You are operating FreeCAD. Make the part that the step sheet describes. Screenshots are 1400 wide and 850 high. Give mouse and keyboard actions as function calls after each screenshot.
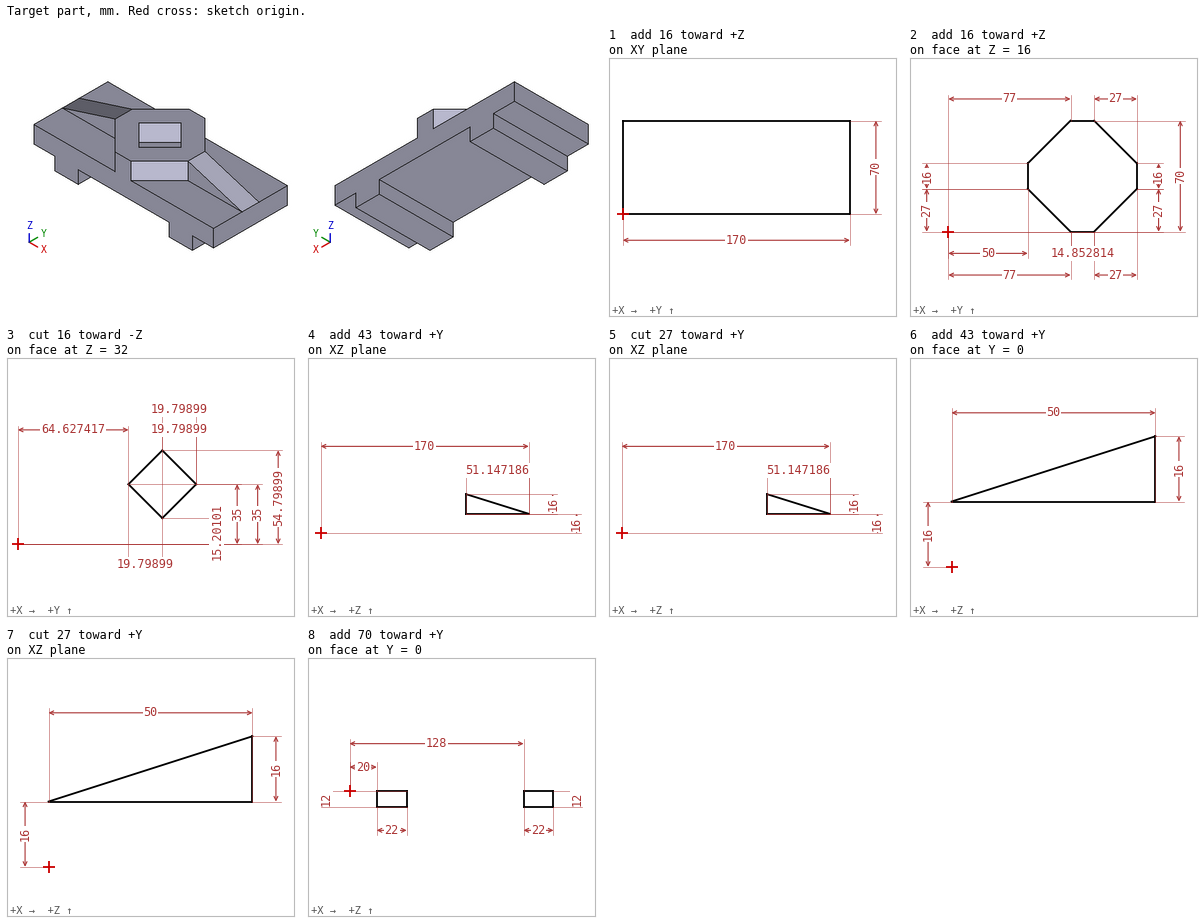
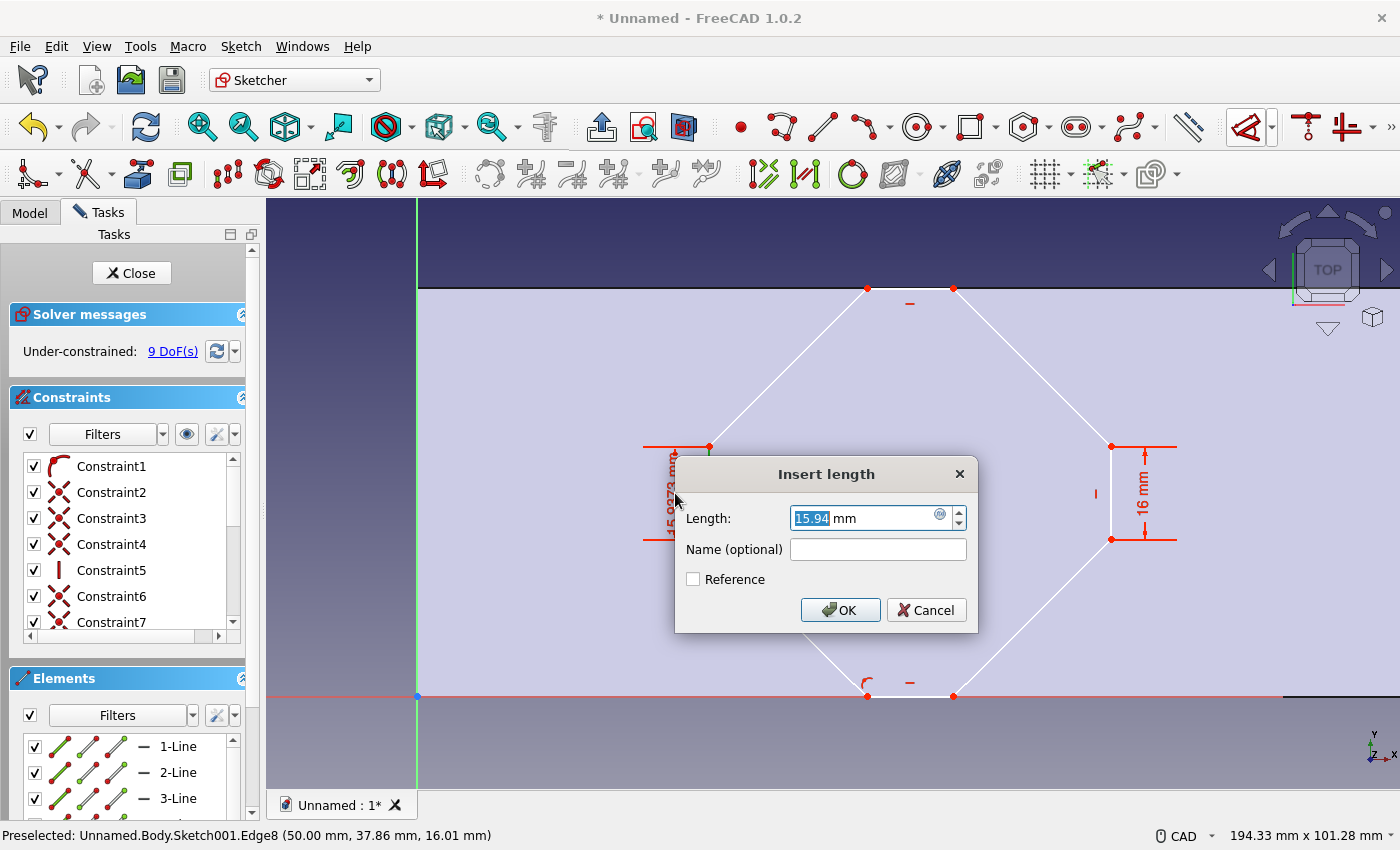
text(16)
key(Return)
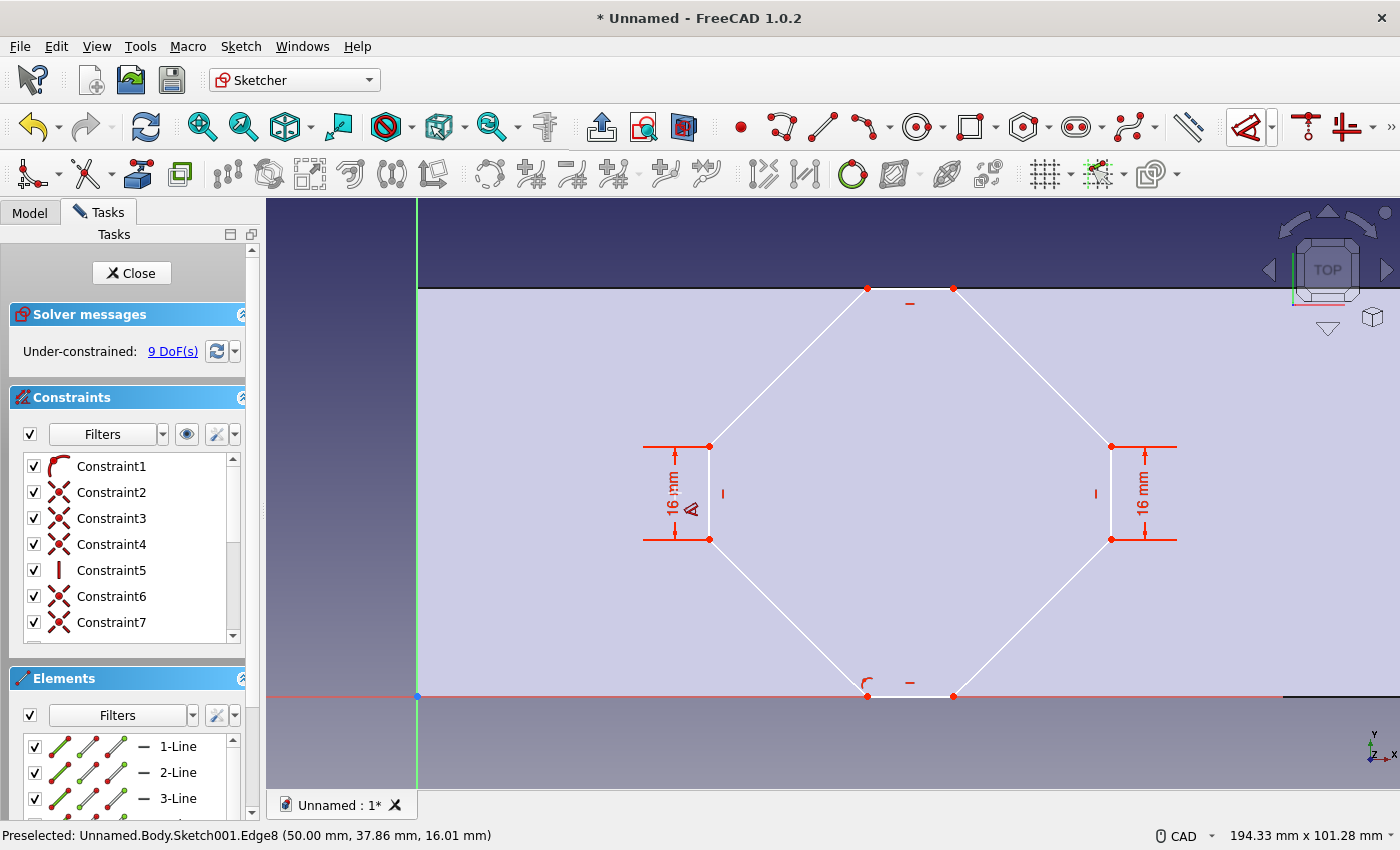
click(709, 540)
click(563, 731)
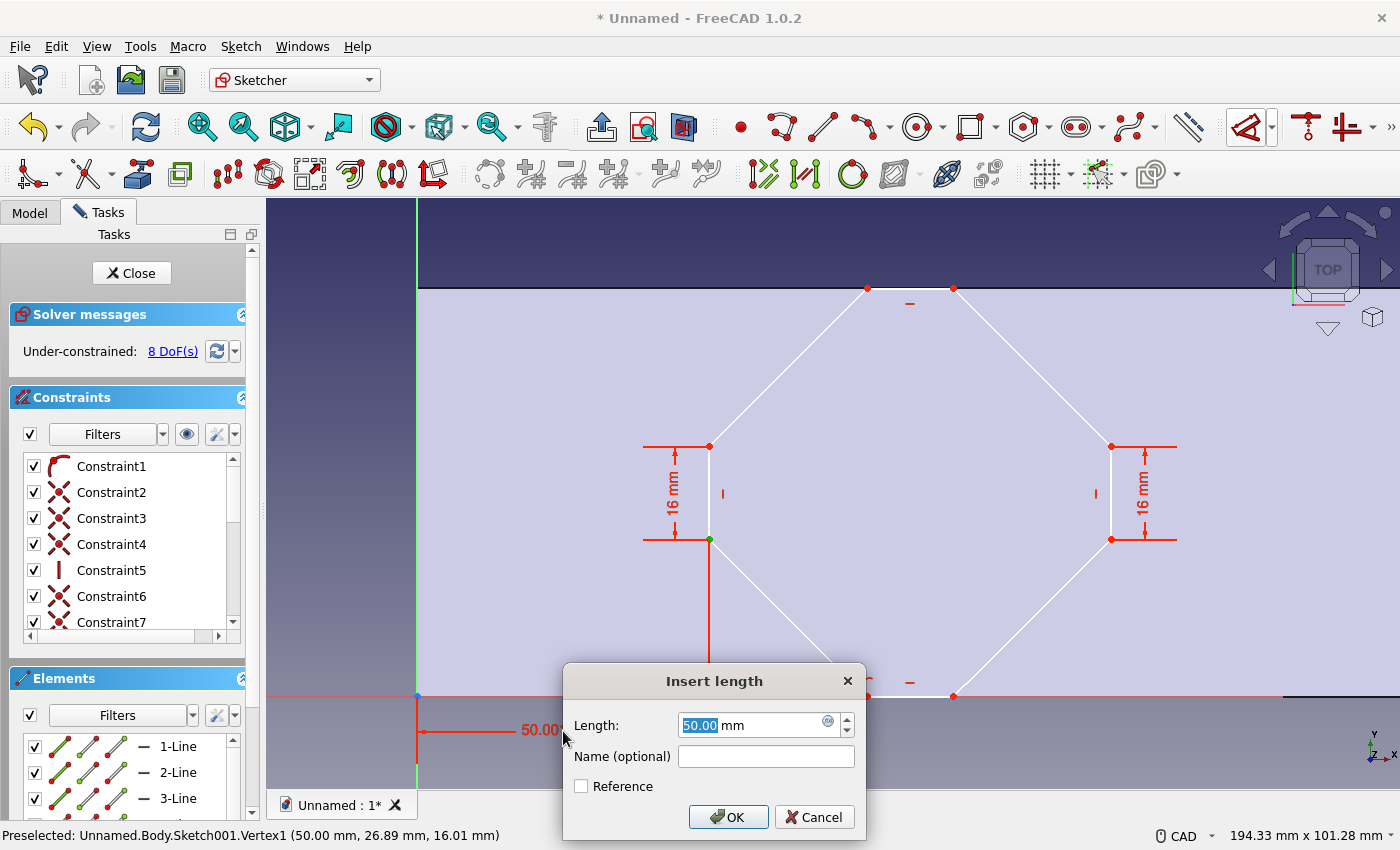
text(50)
key(Return)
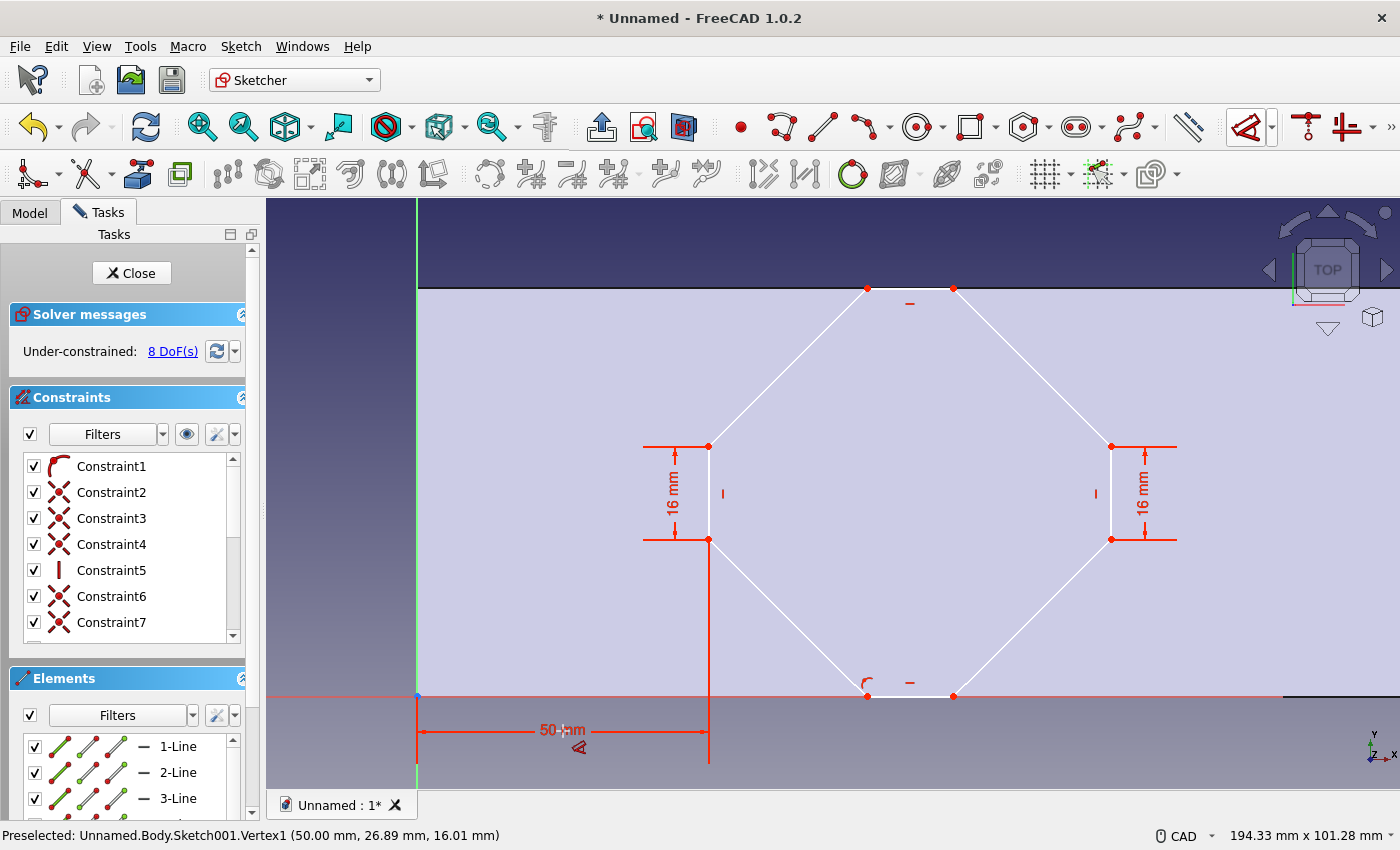
click(709, 540)
click(383, 618)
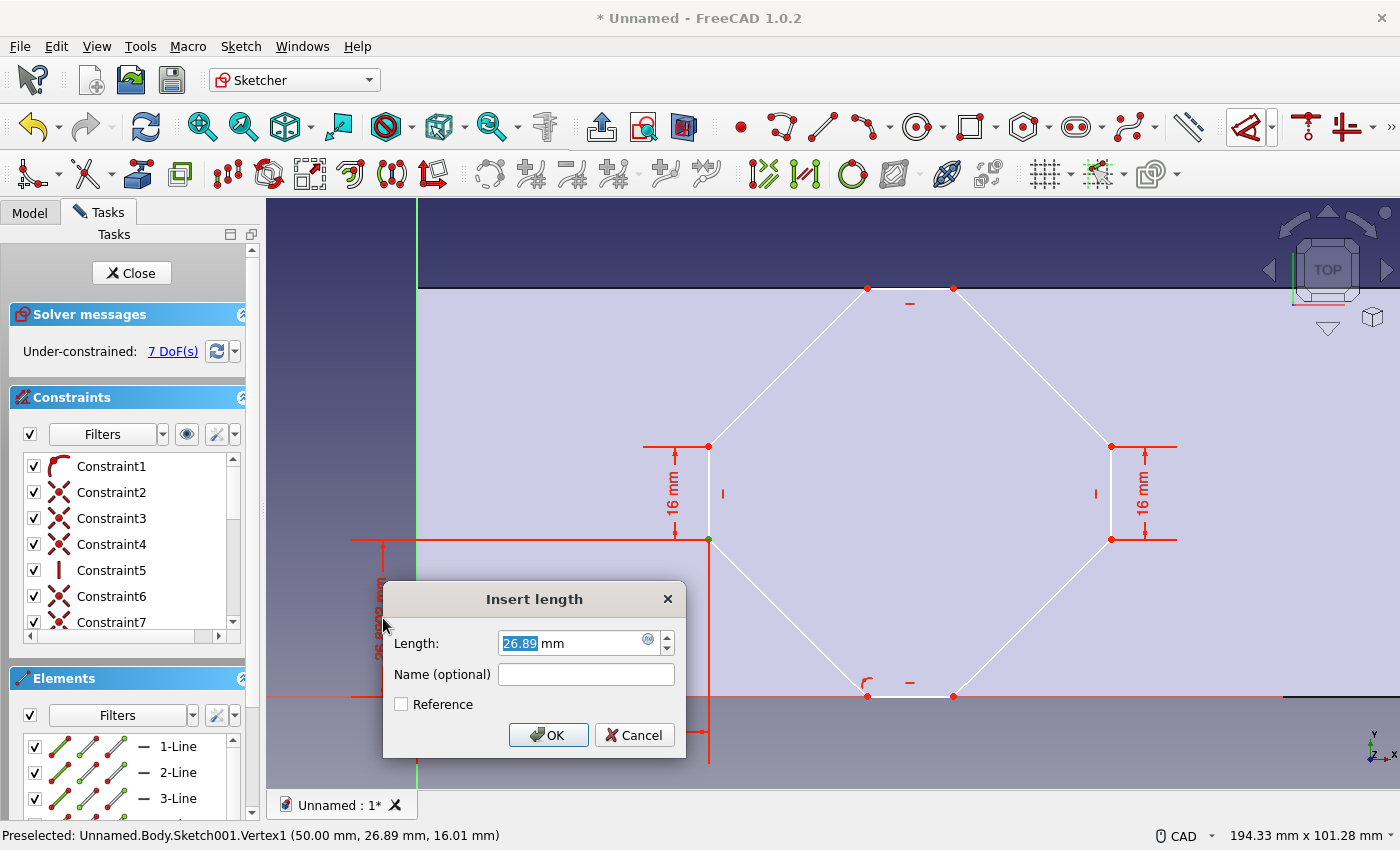
text(27)
key(Return)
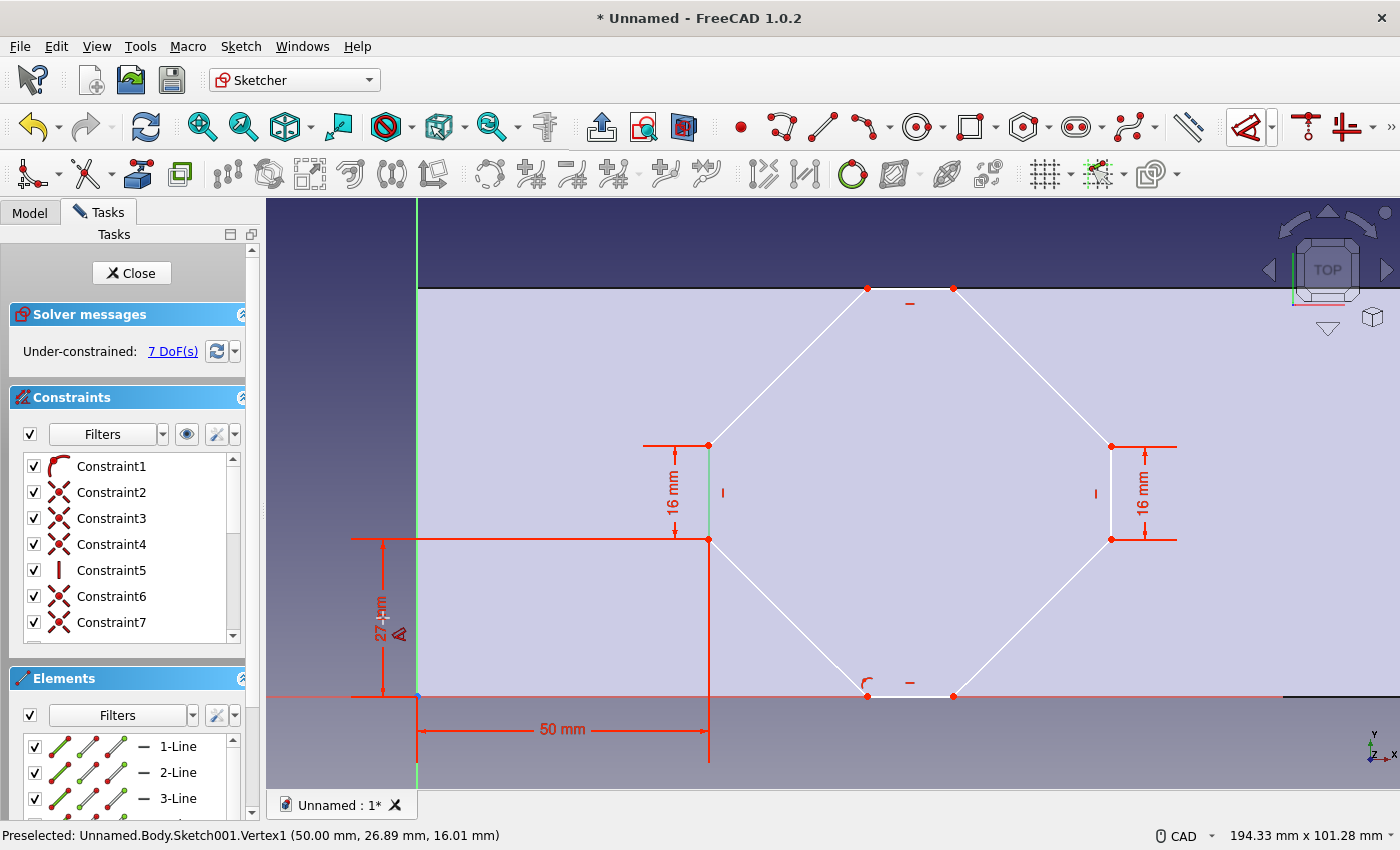
click(867, 697)
click(642, 731)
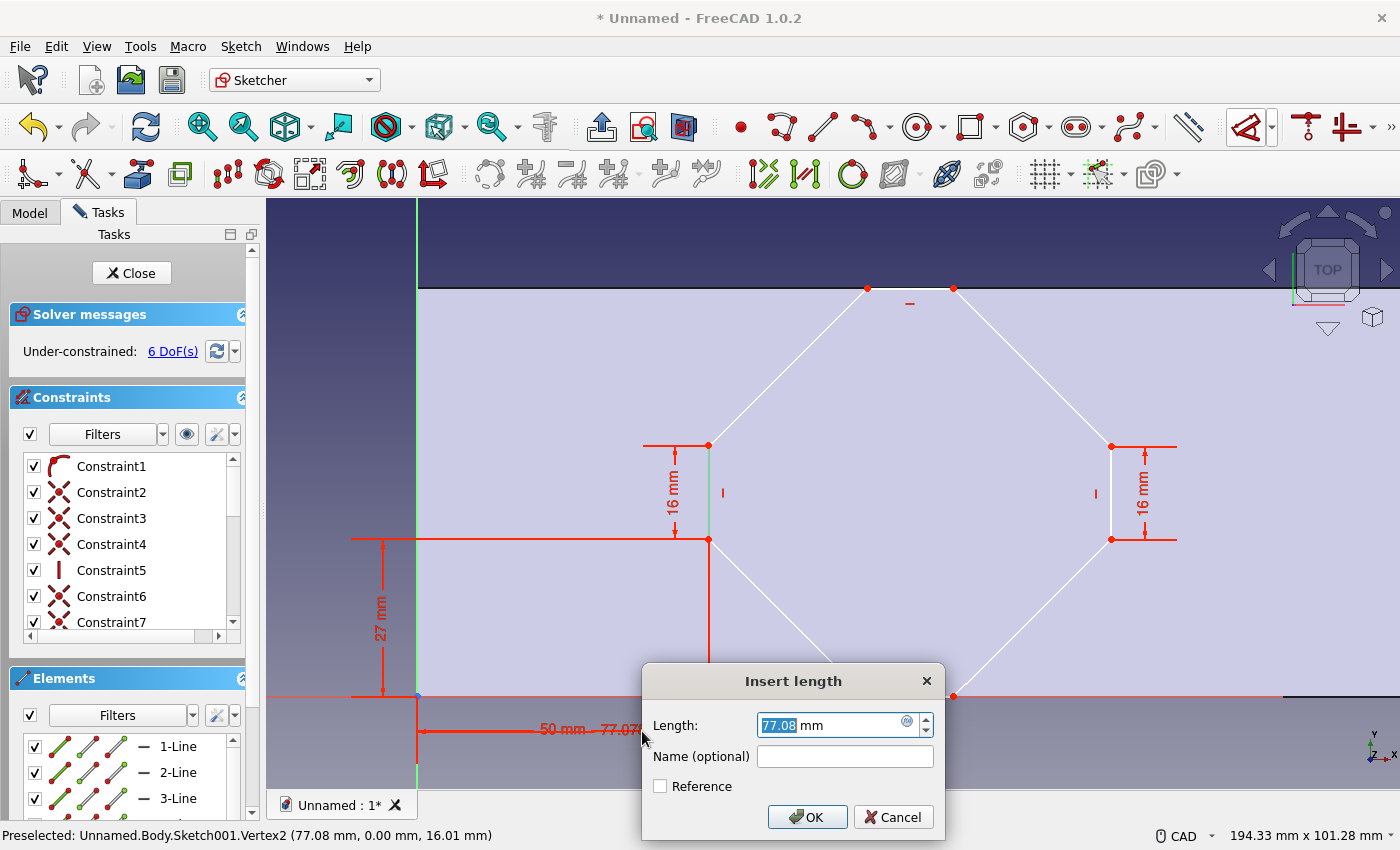
text(77)
key(Return)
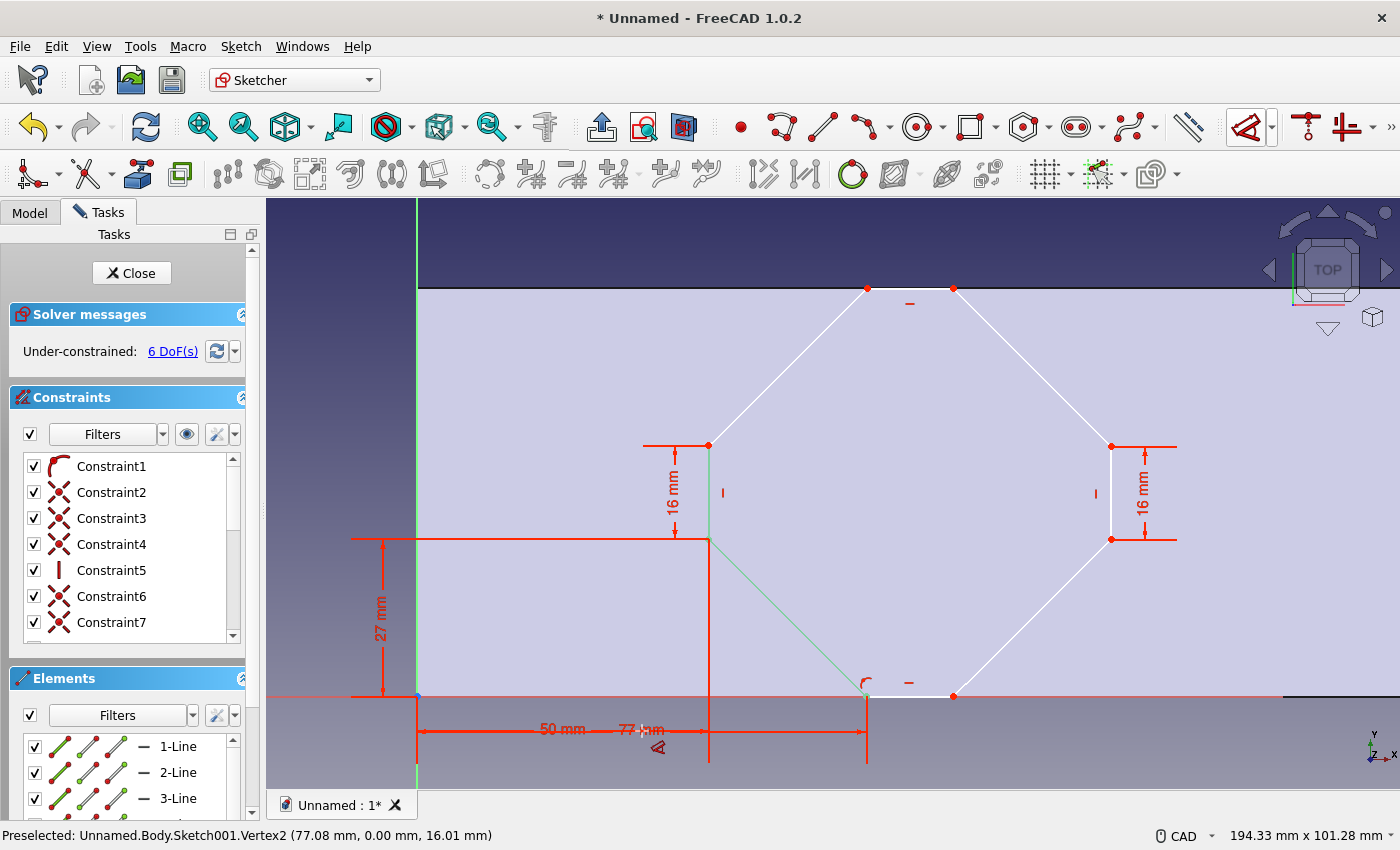
click(1111, 540)
click(1145, 618)